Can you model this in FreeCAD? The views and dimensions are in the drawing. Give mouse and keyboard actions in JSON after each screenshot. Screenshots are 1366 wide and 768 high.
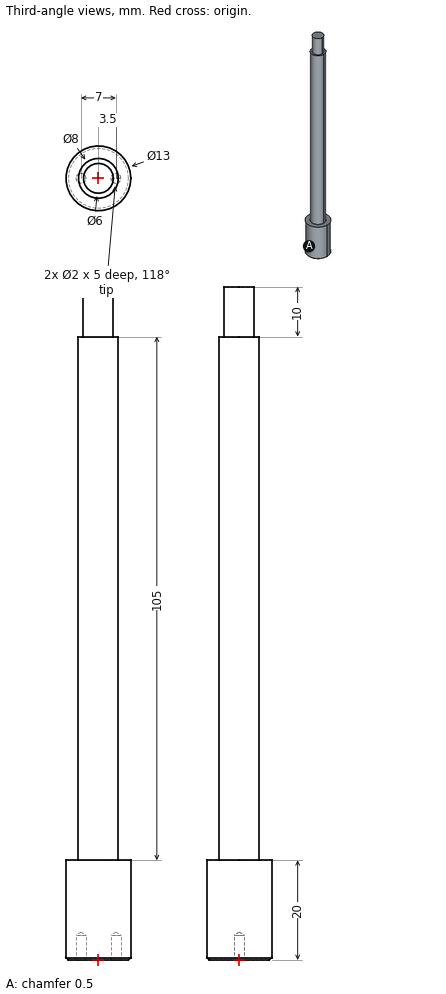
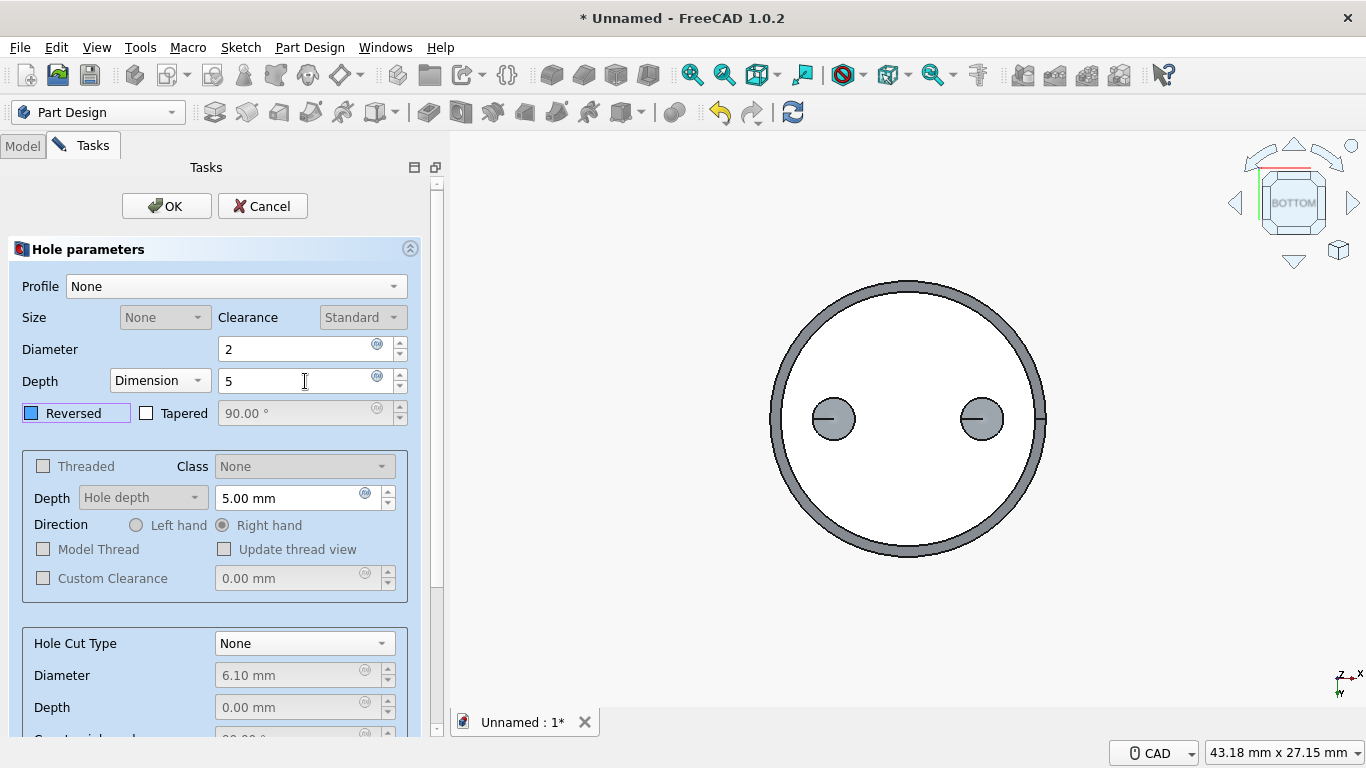
{"action": "left_click", "coordinate": [167, 206]}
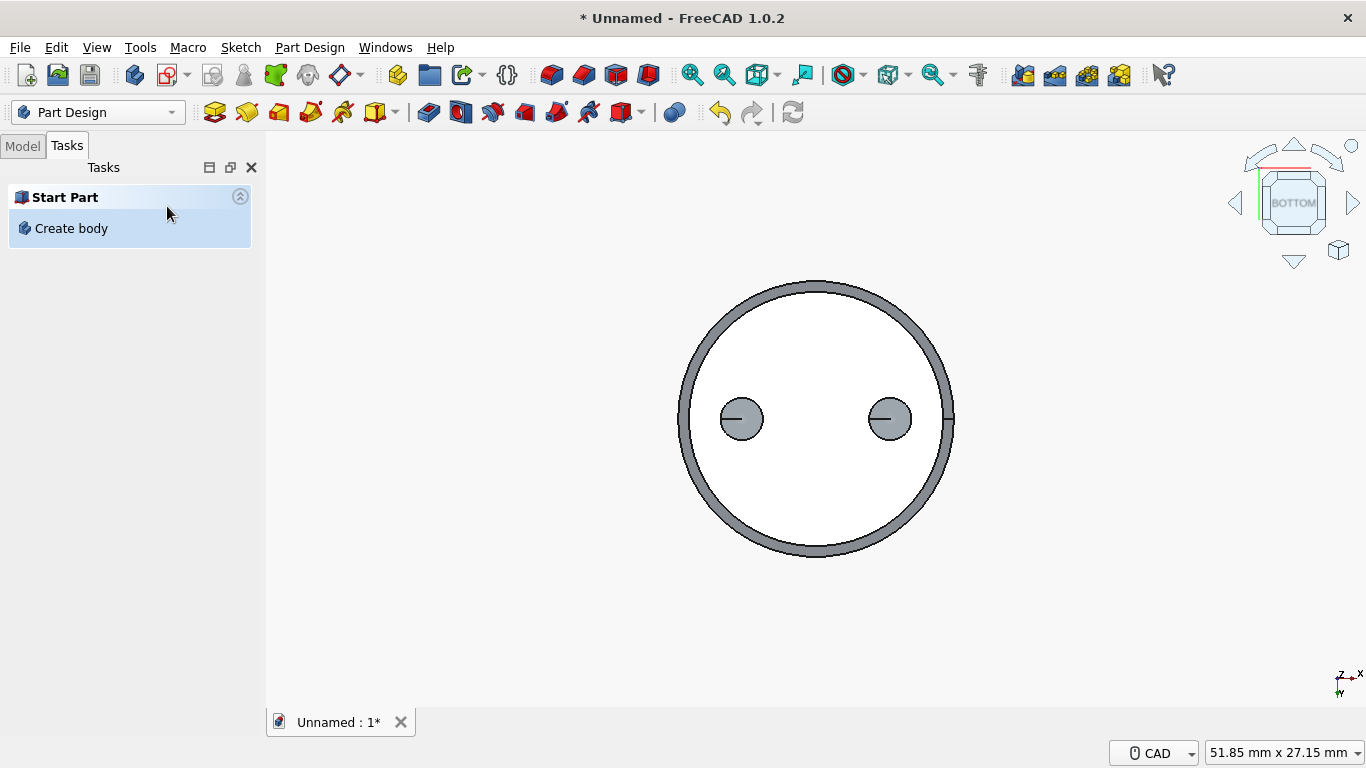
{"action": "key", "text": "0"}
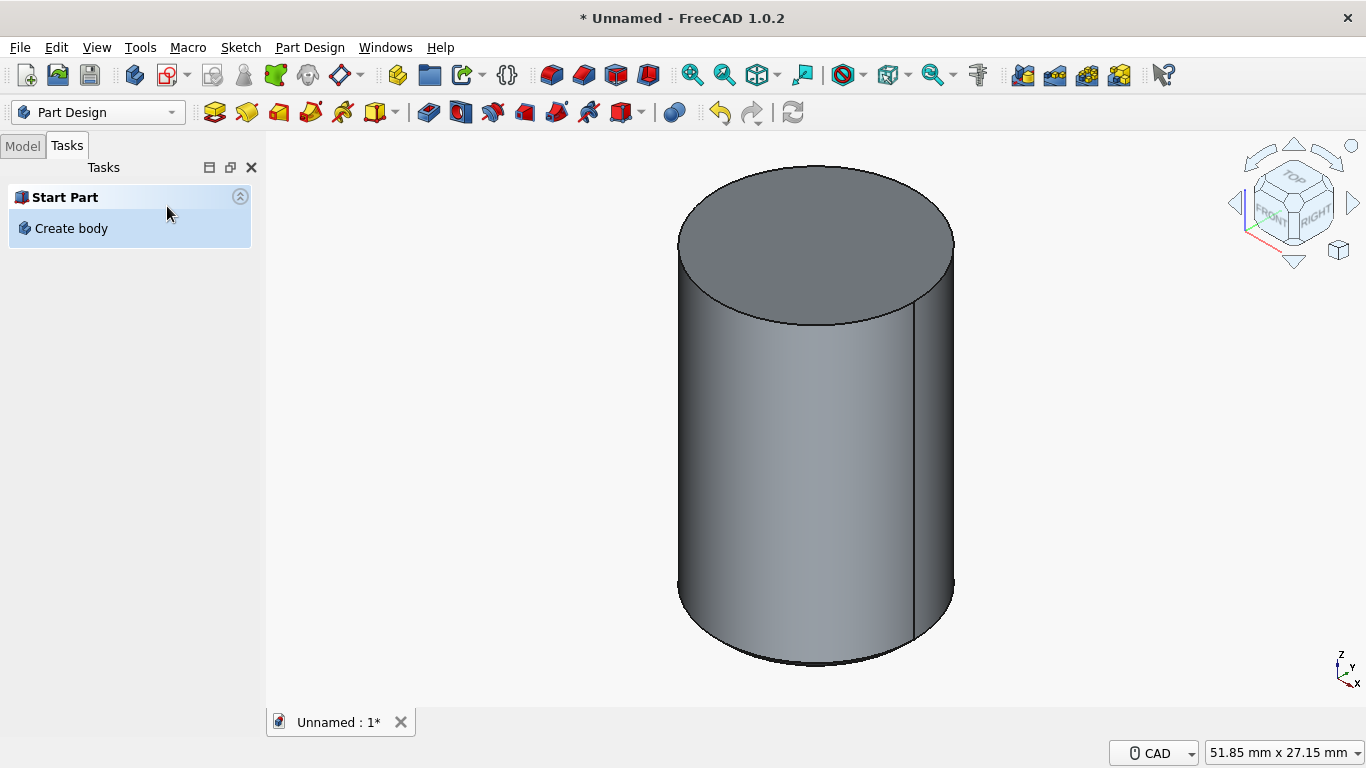
{"action": "left_click", "coordinate": [816, 245]}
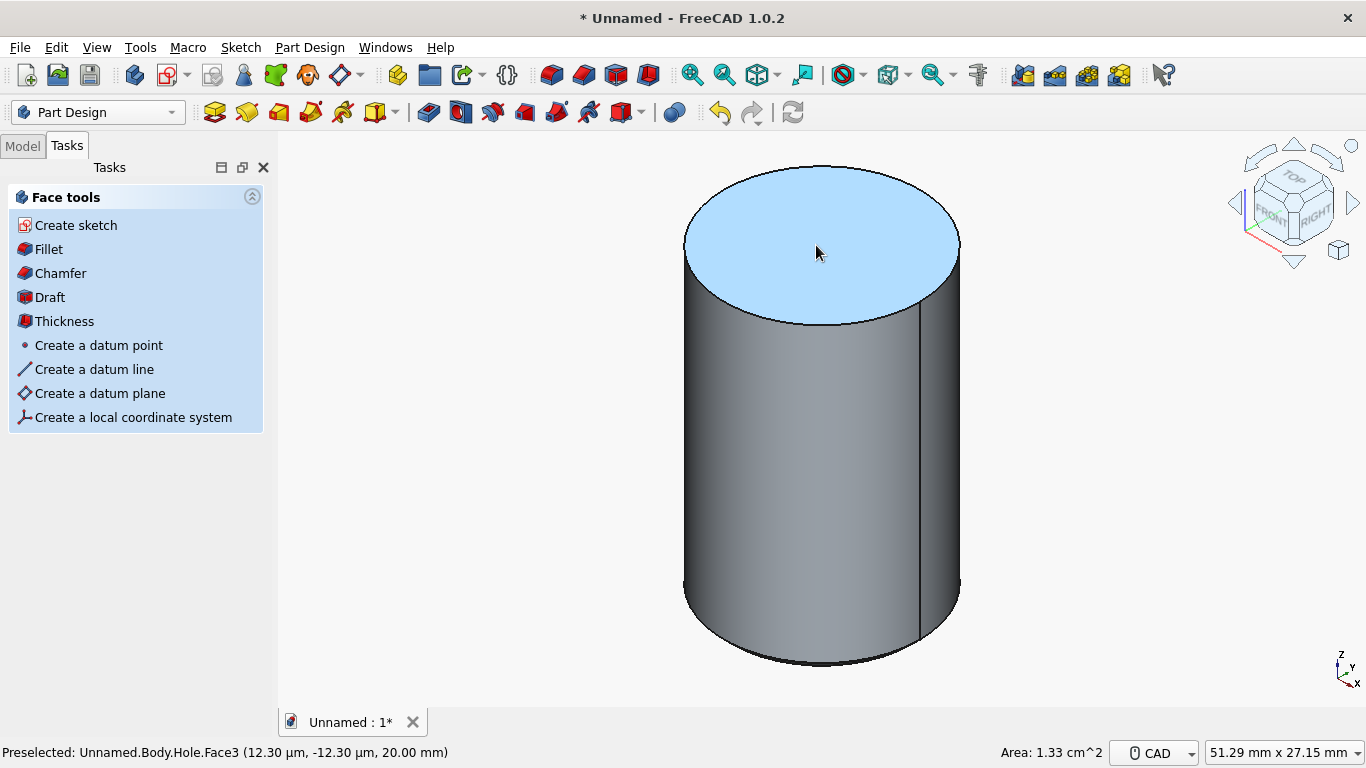
{"action": "left_click", "coordinate": [168, 76]}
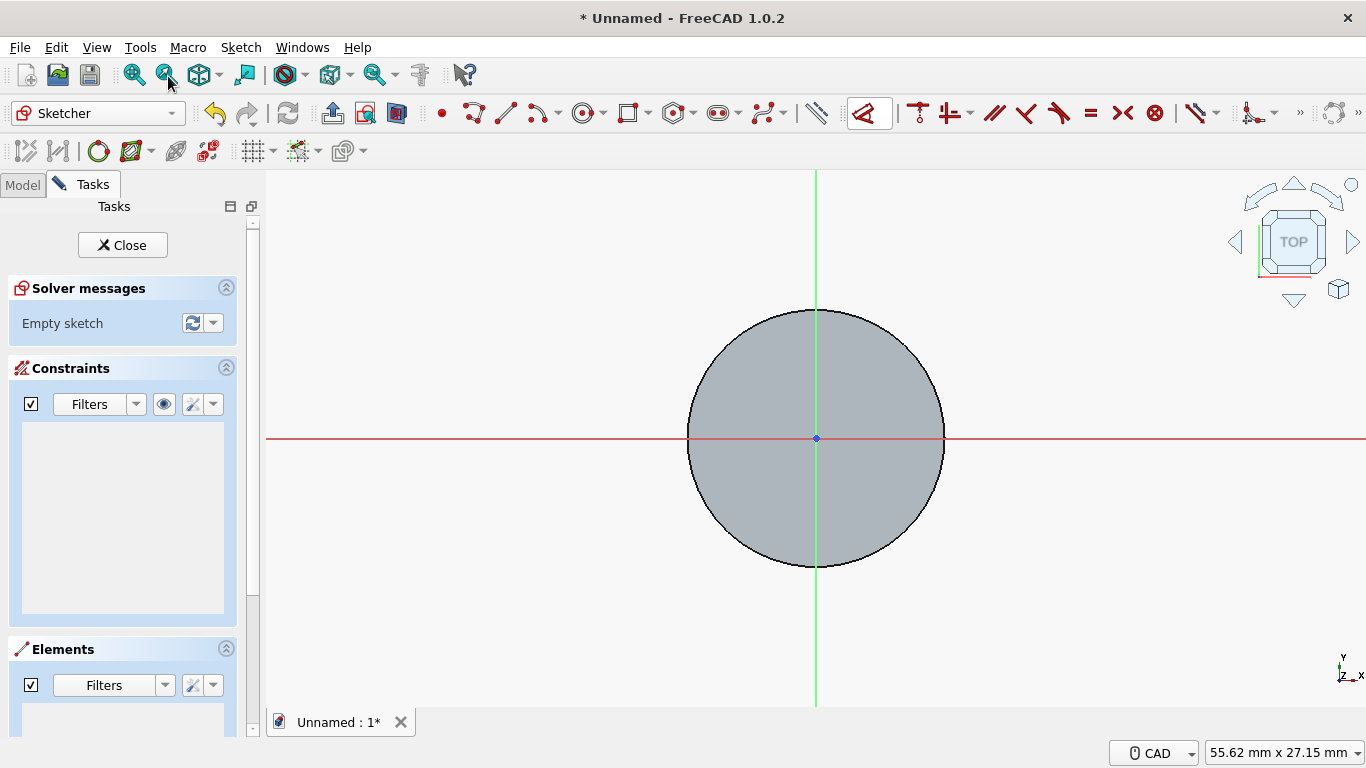
{"action": "scroll", "coordinate": [872, 438], "scroll_direction": "up", "scroll_amount": 4}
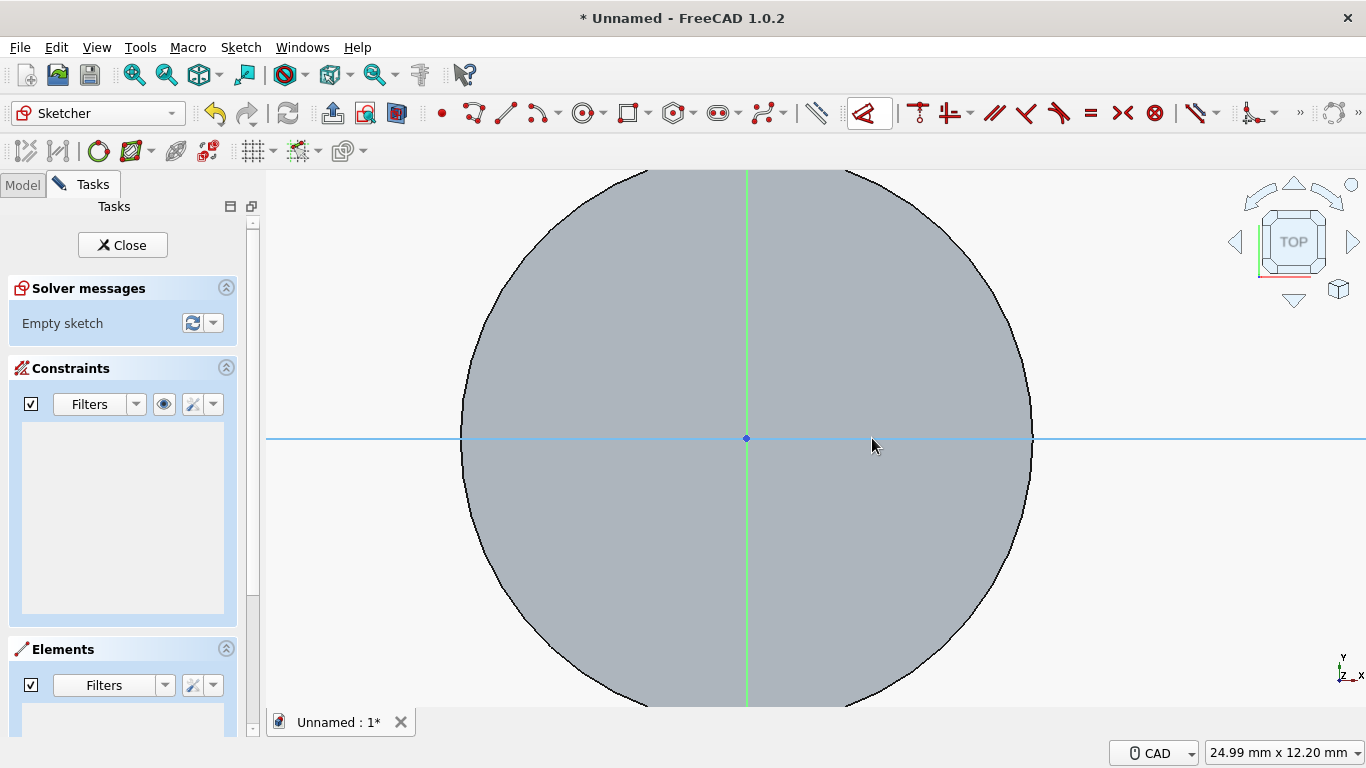
{"action": "key", "text": "g c"}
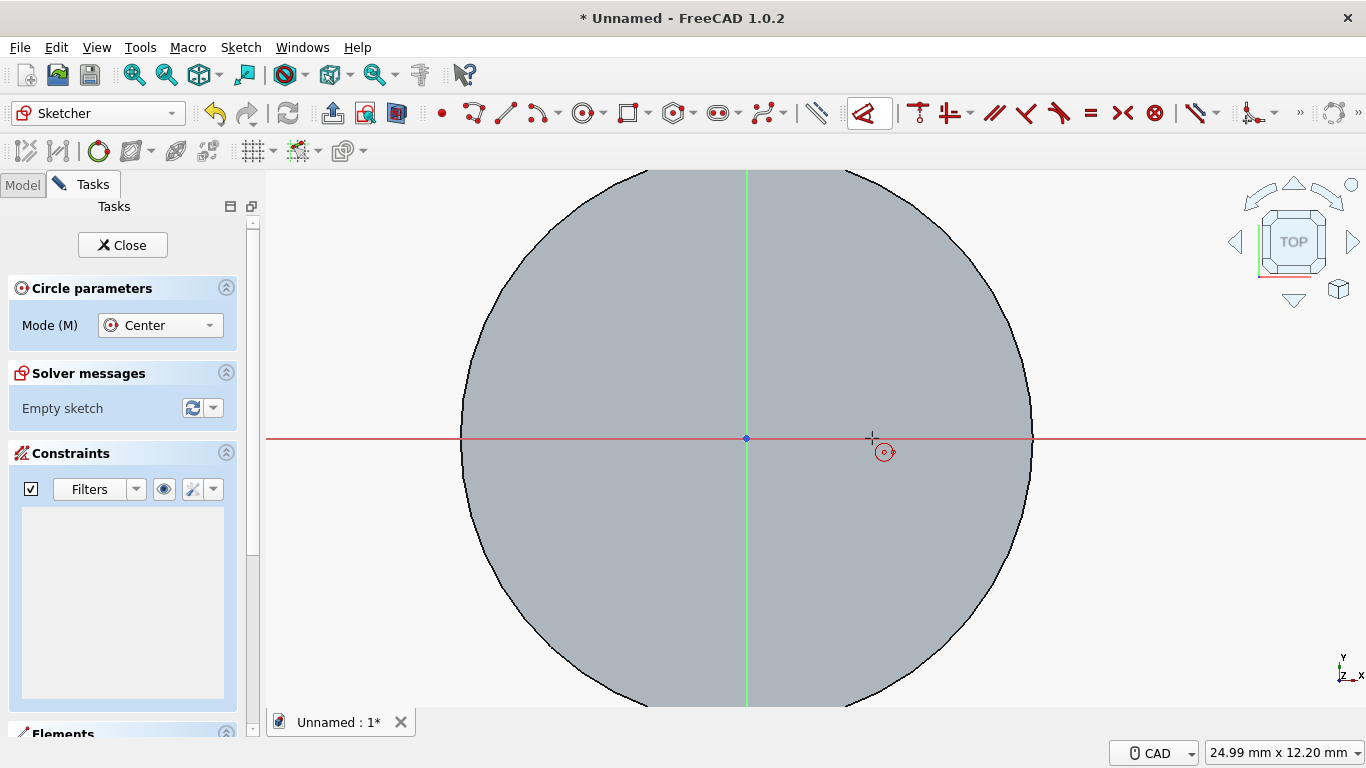
{"action": "left_click", "coordinate": [747, 438]}
{"action": "left_click", "coordinate": [871, 314]}
{"action": "key", "text": "Escape"}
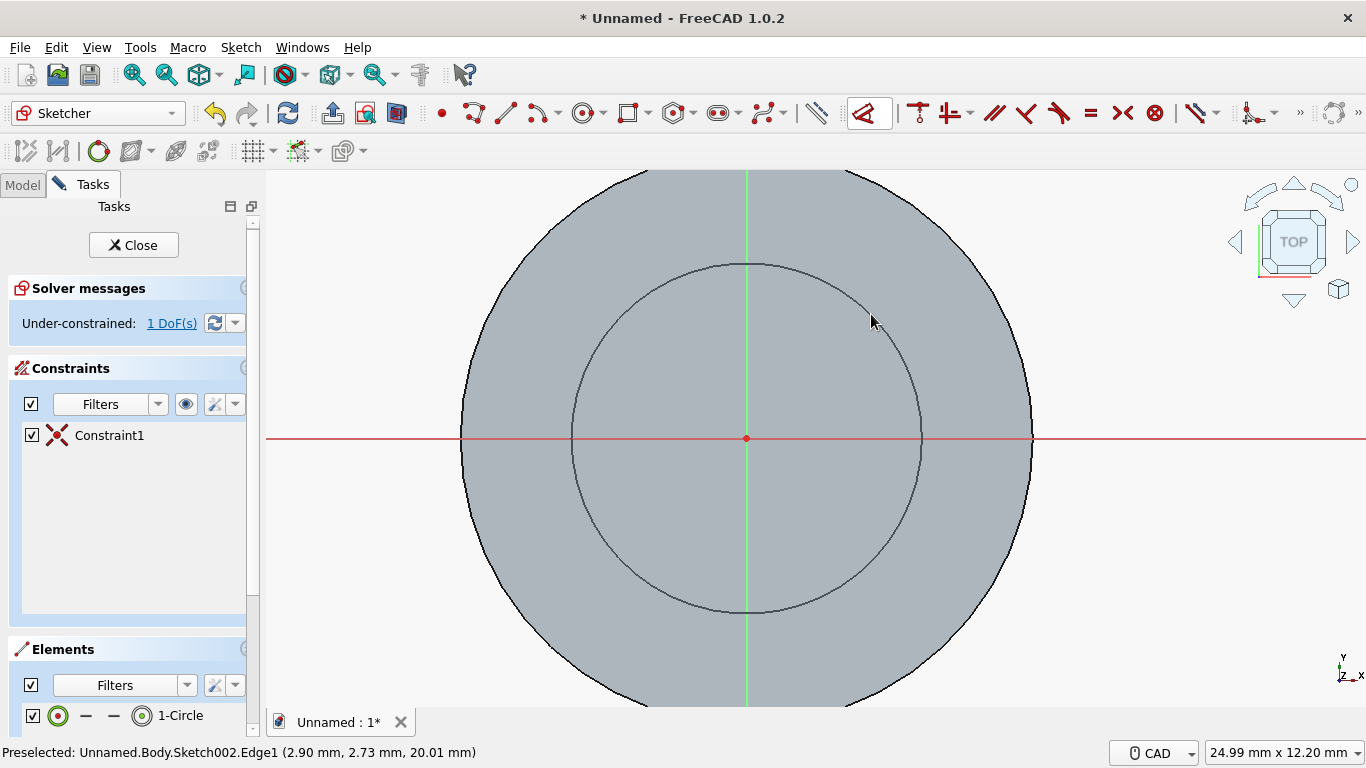
{"action": "left_click", "coordinate": [870, 314]}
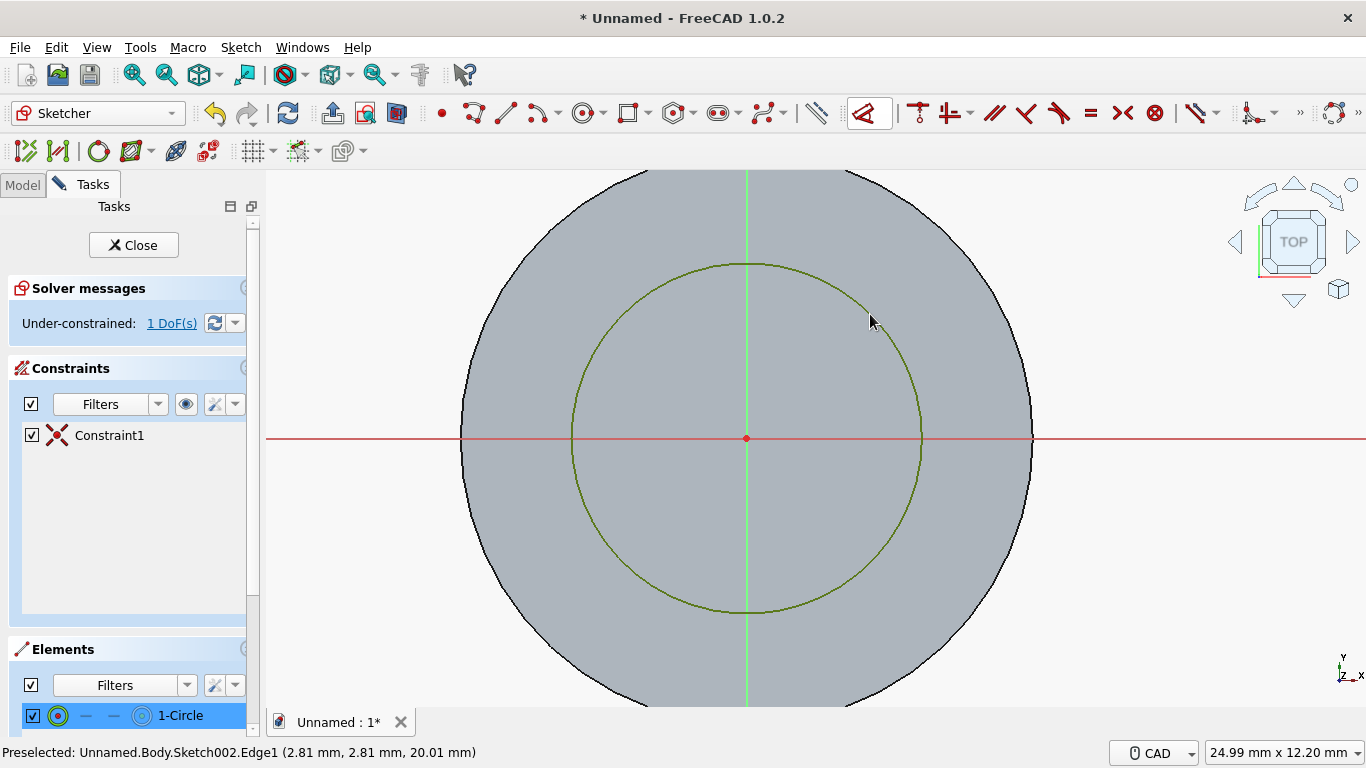
{"action": "left_click", "coordinate": [886, 114]}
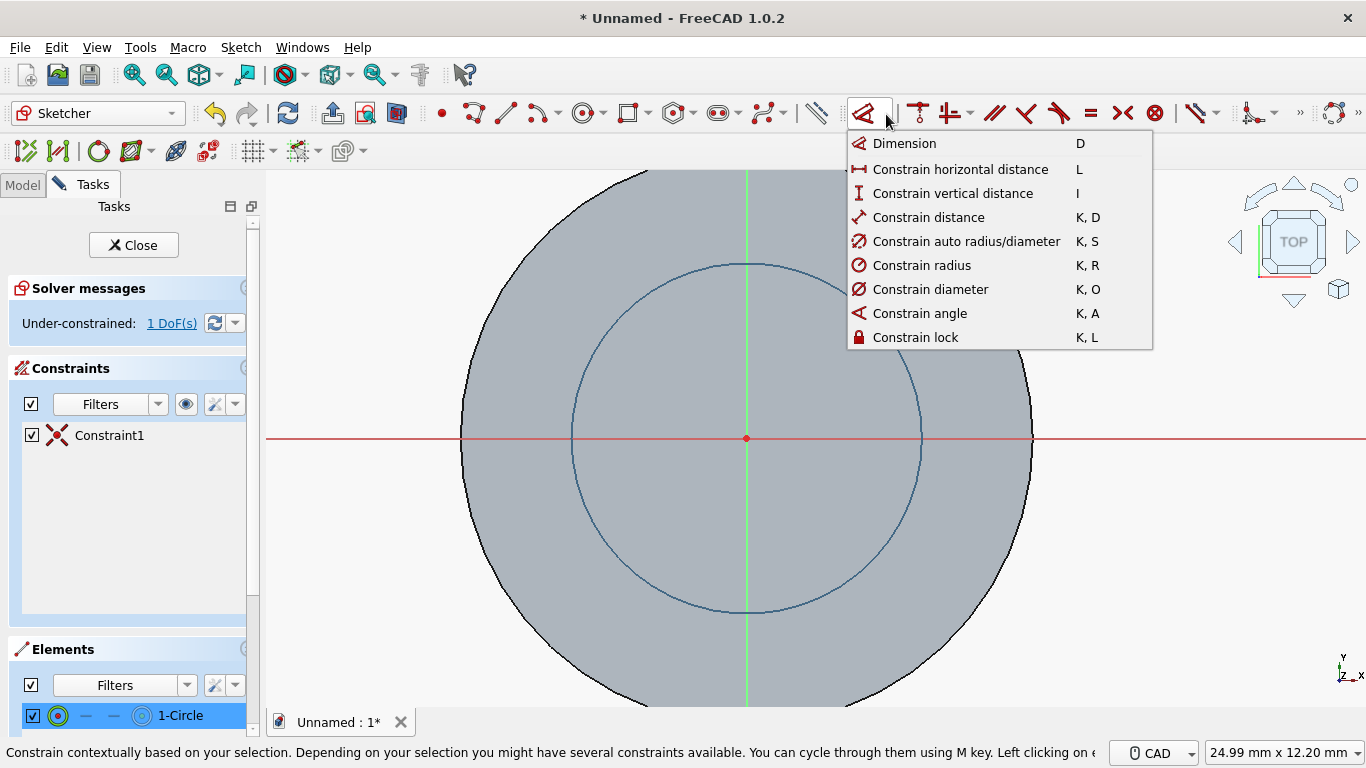
{"action": "left_click", "coordinate": [1000, 289]}